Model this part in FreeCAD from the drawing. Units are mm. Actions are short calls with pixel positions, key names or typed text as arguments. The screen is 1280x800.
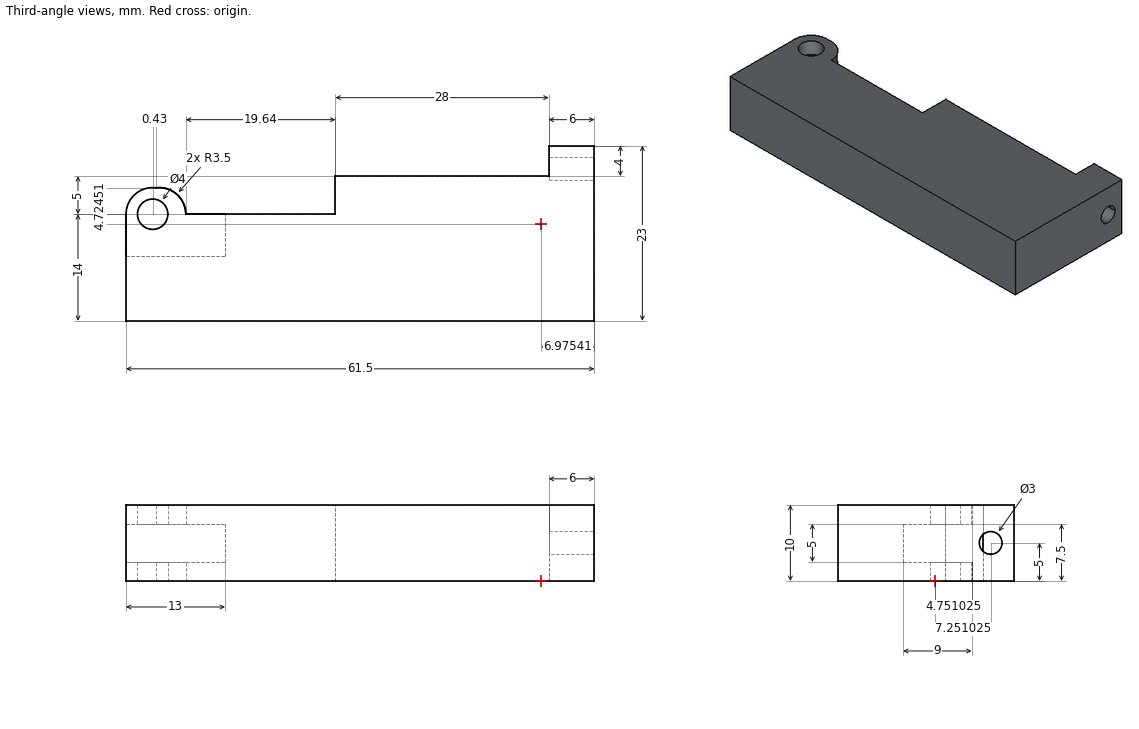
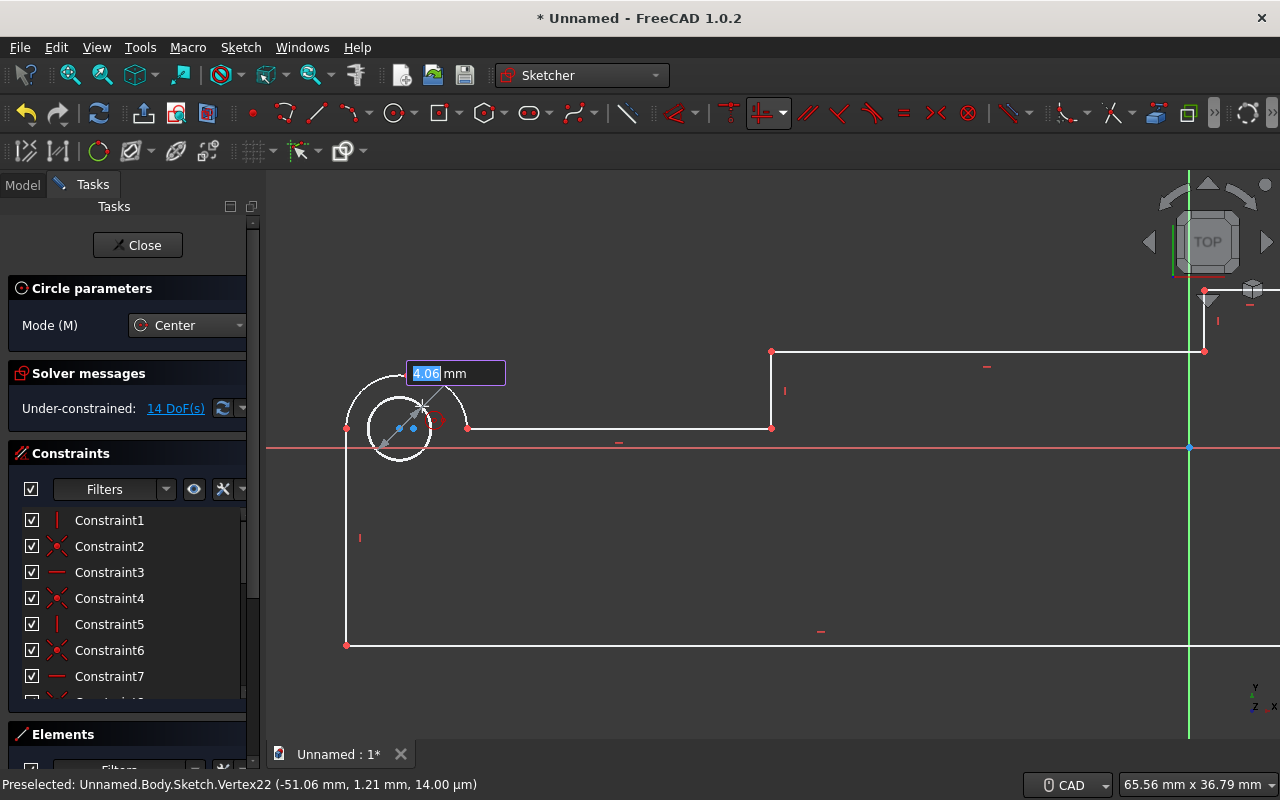
text(4)
key(Return)
key(Escape)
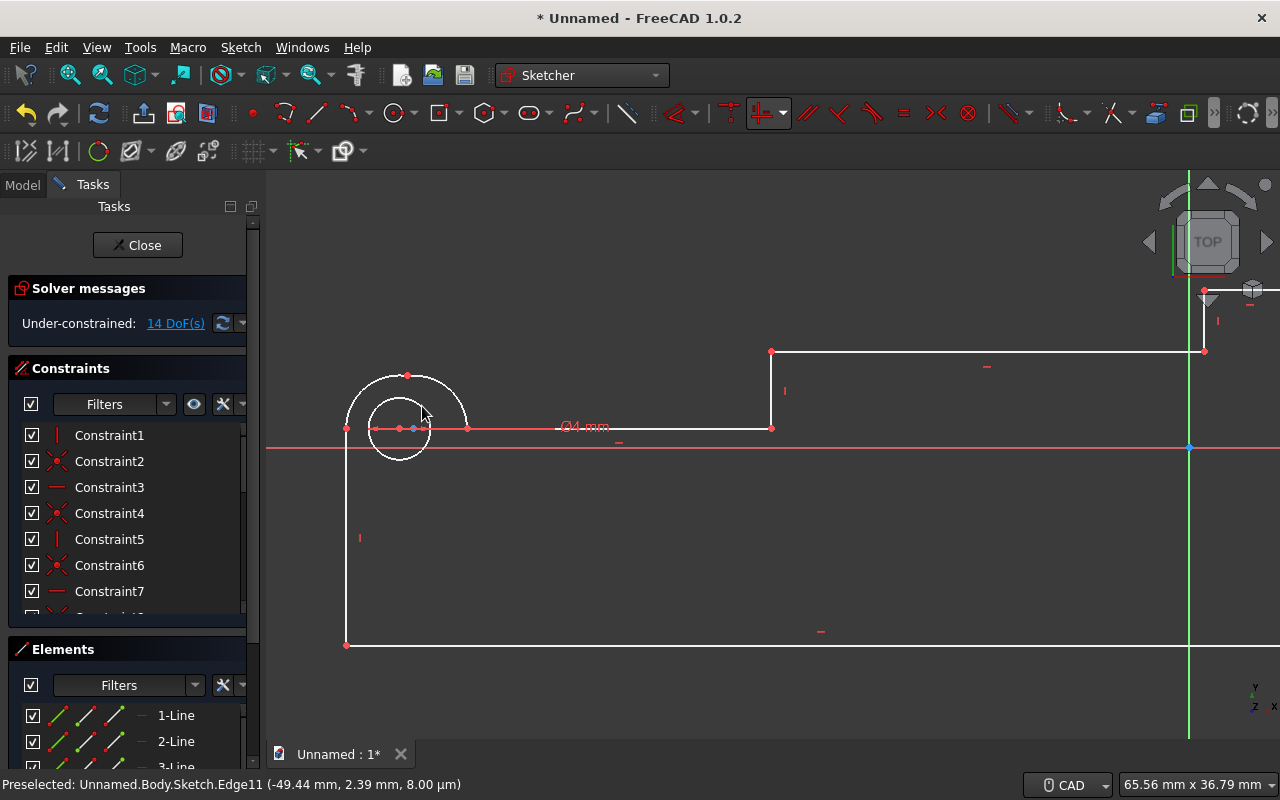
click(346, 494)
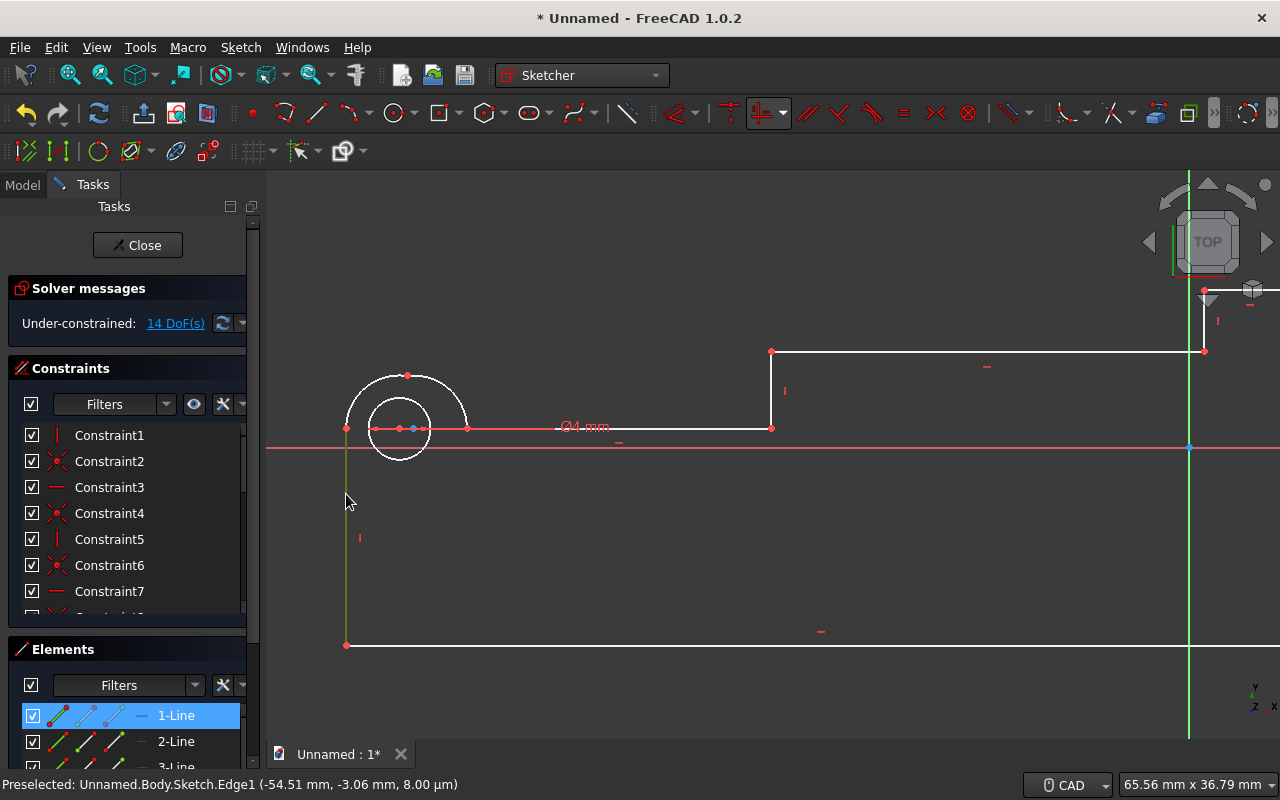
click(380, 379)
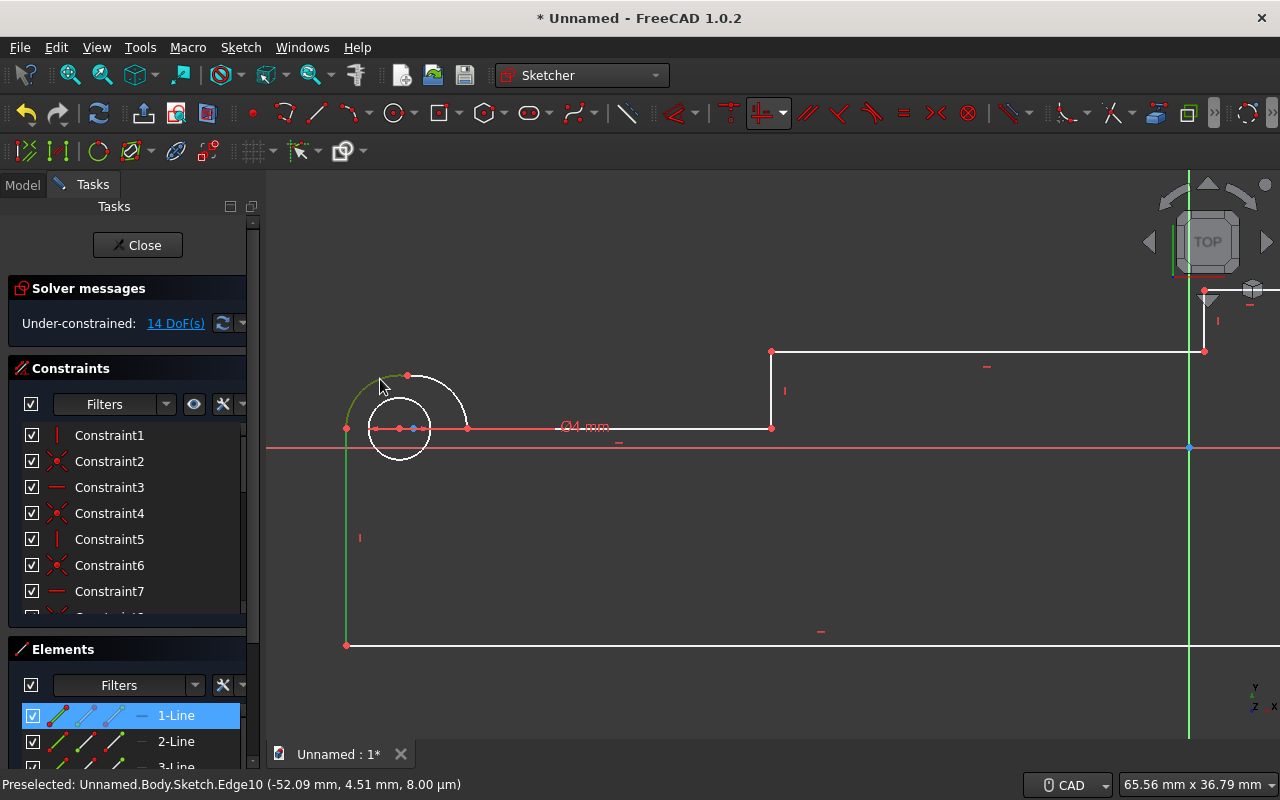
key(t)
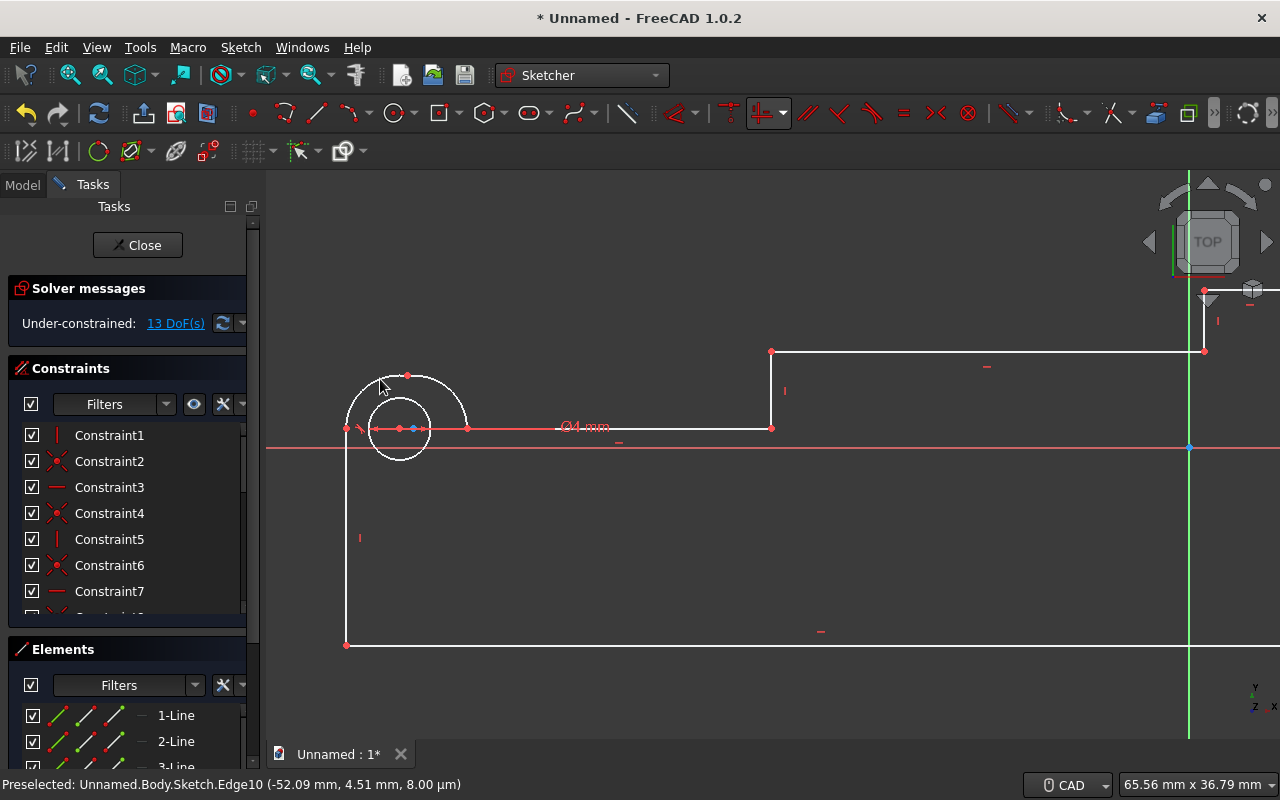
click(460, 403)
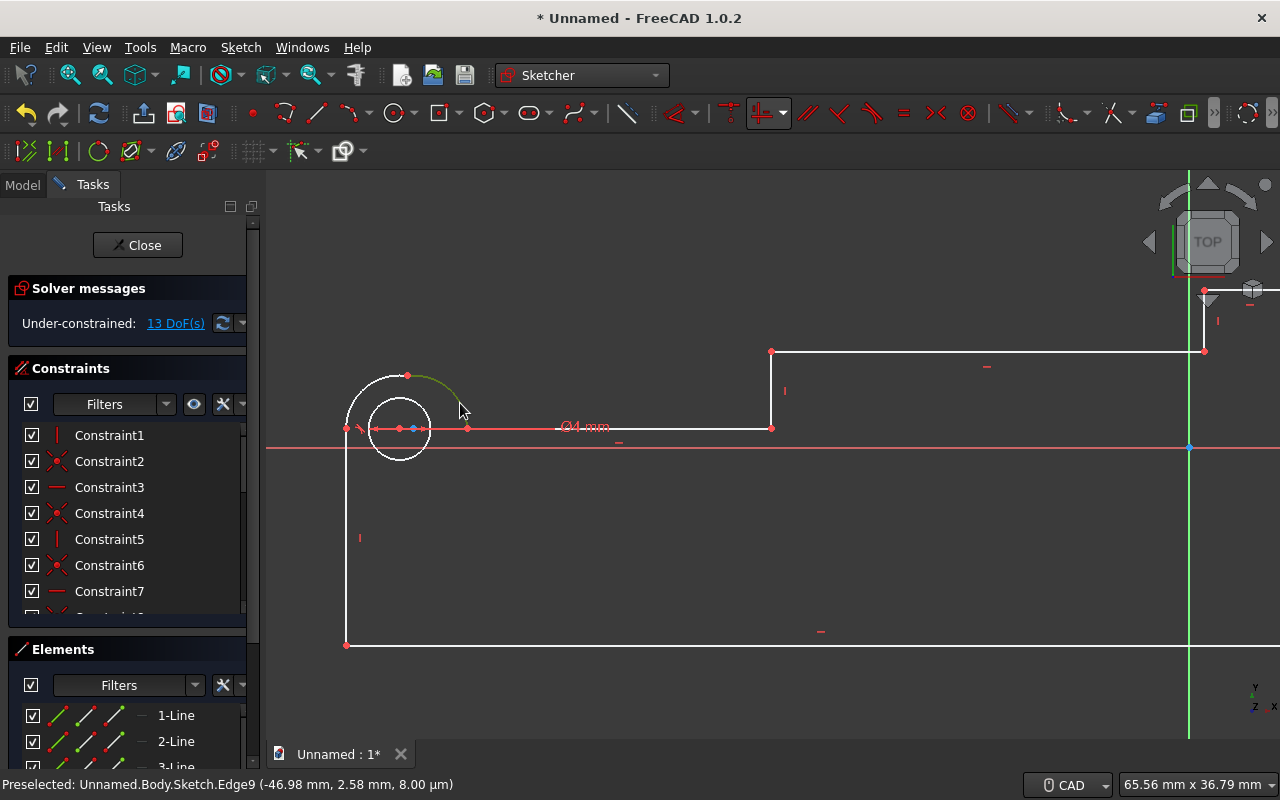
click(380, 379)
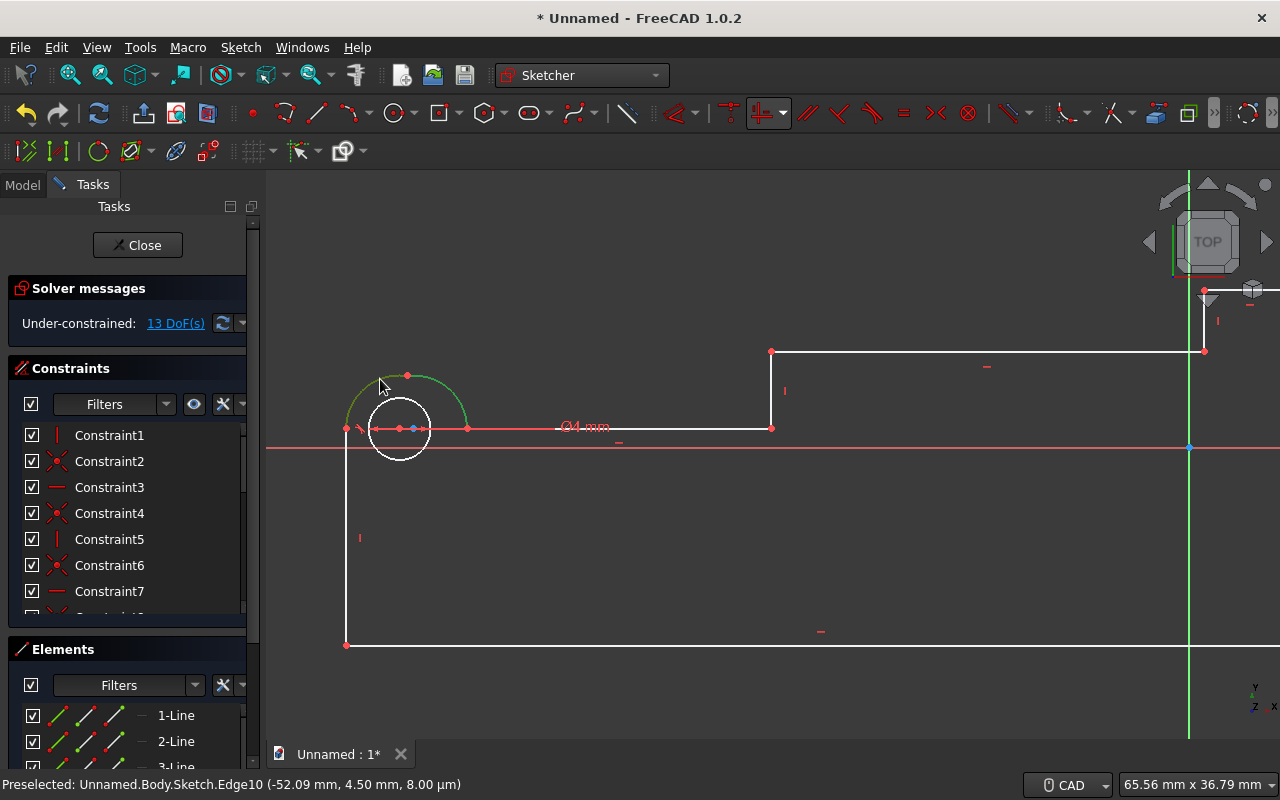
key(e)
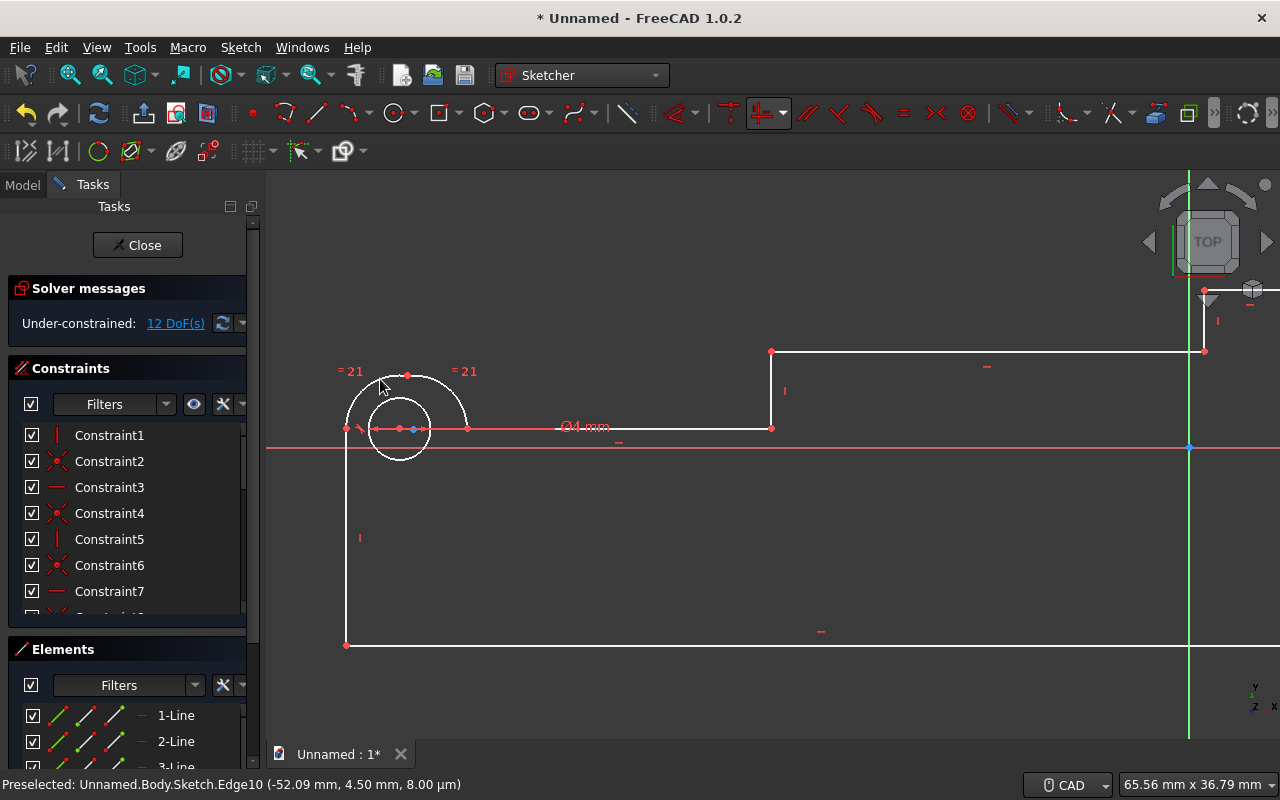
key(d)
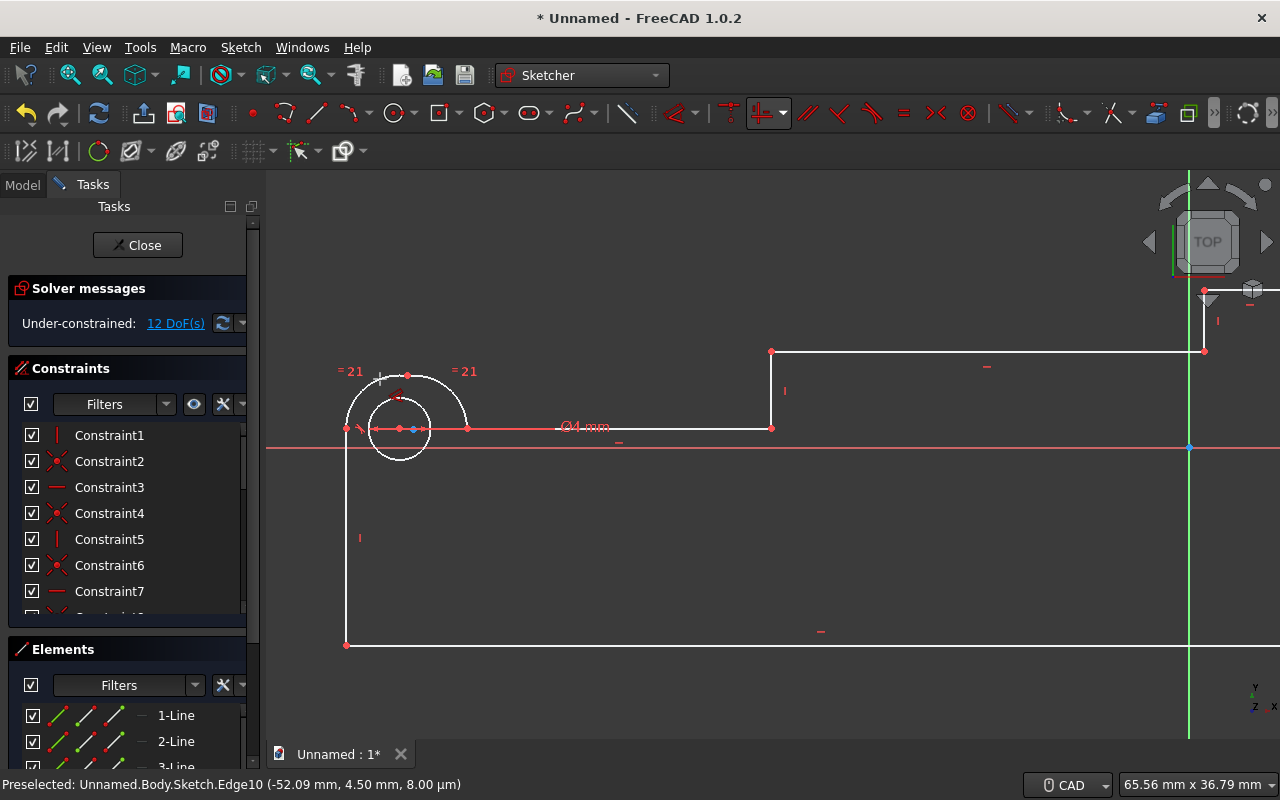
click(460, 403)
click(488, 387)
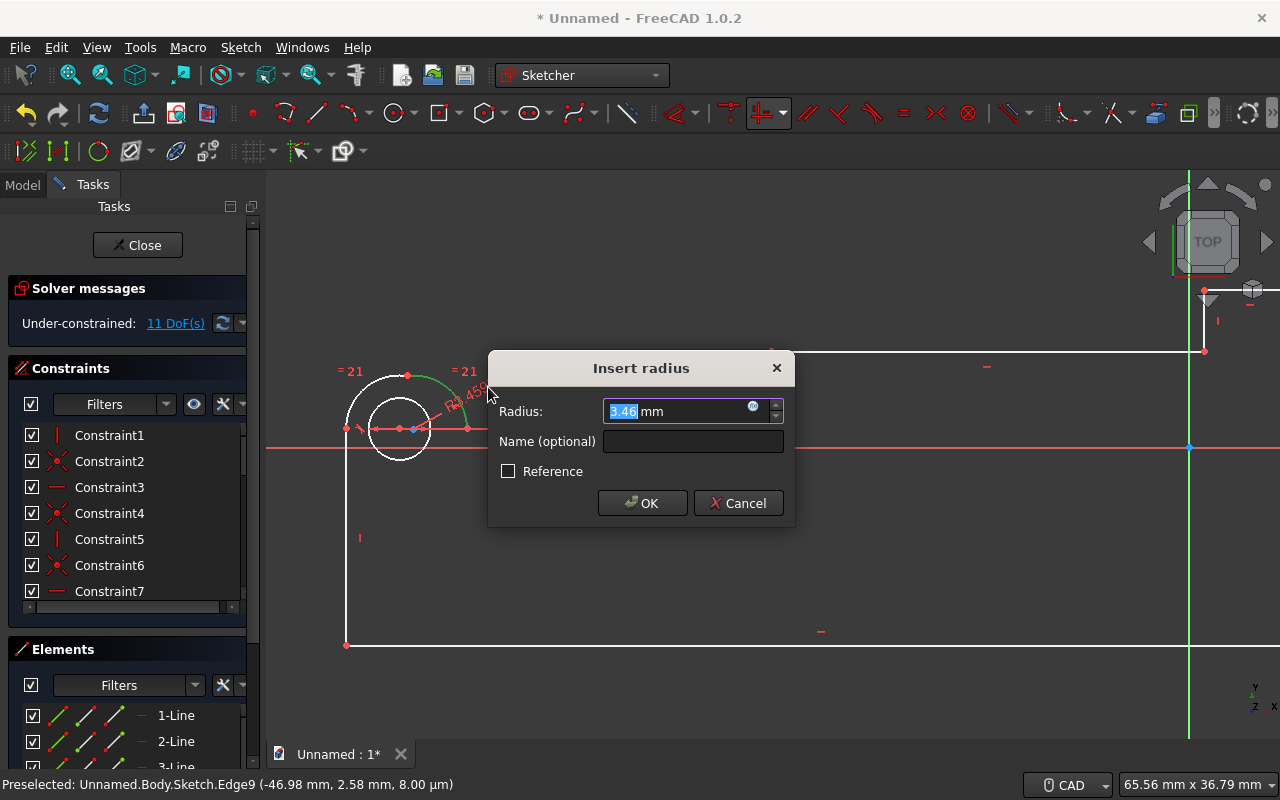
text(3.5)
key(Return)